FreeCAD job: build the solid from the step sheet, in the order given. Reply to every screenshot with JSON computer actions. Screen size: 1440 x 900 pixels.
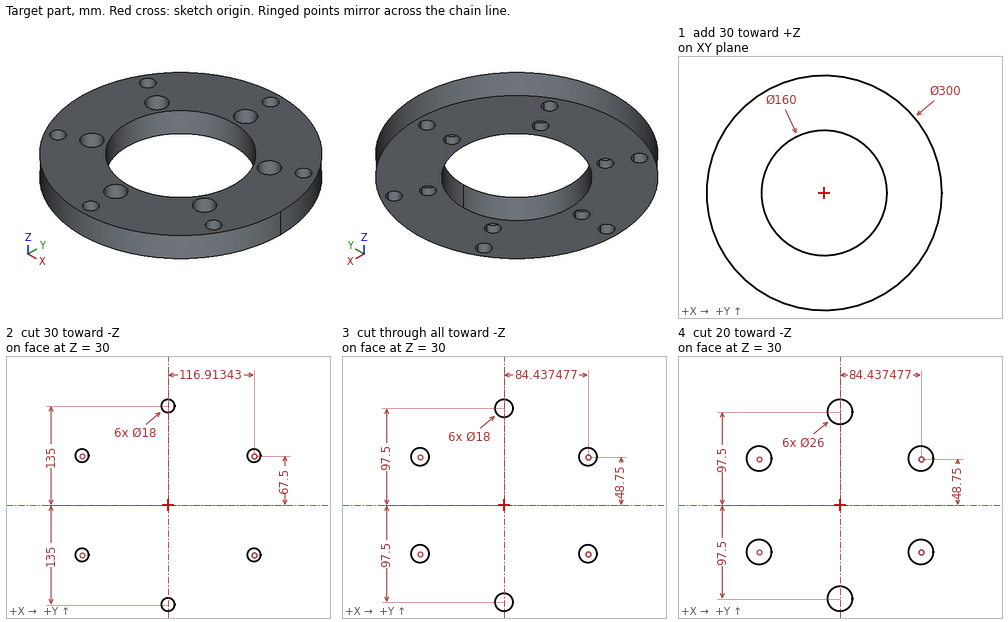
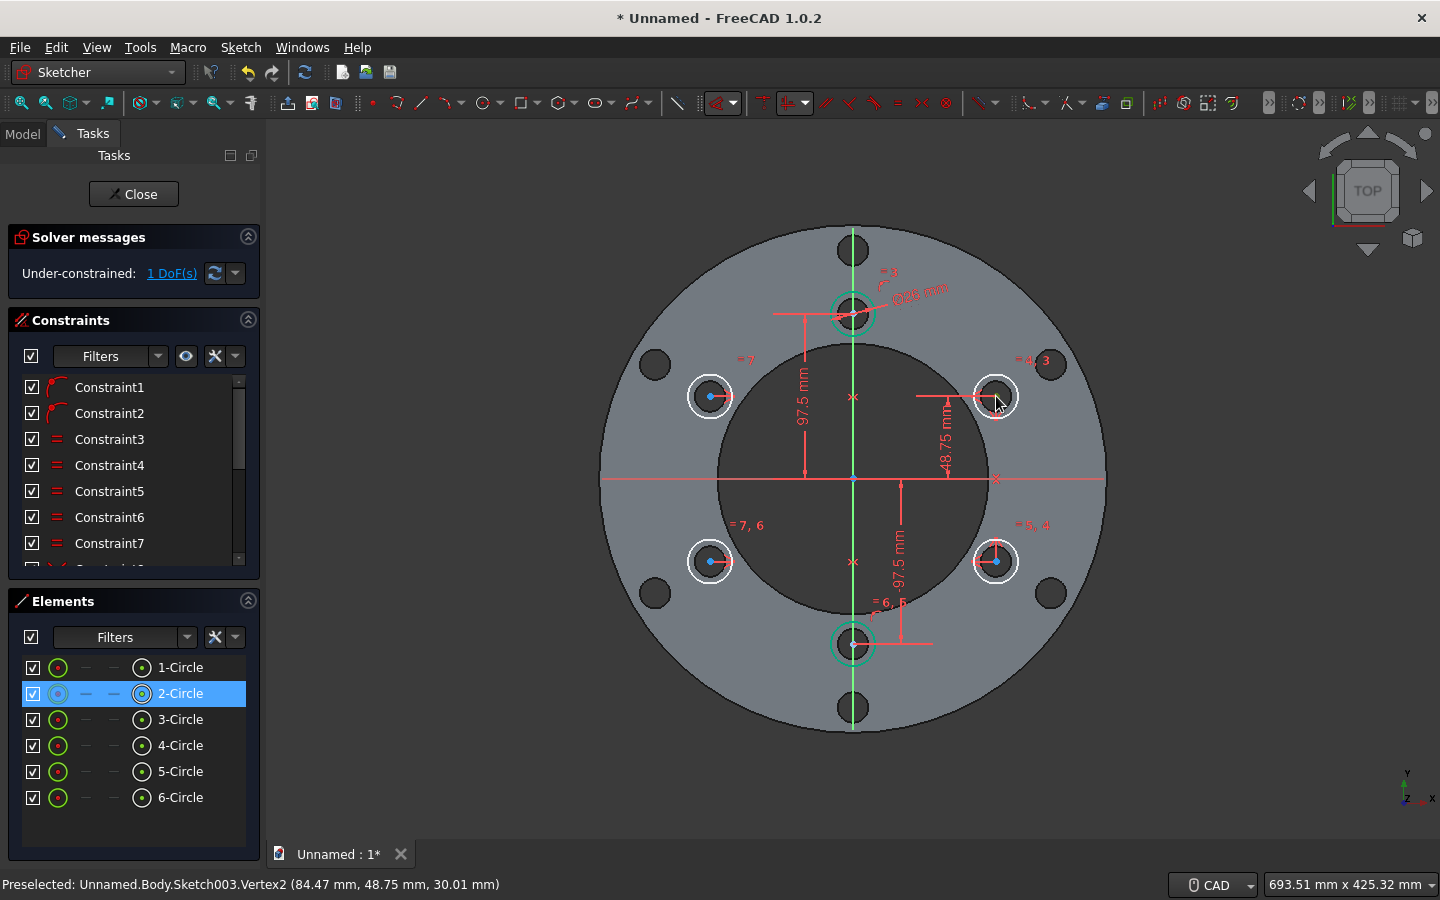
{"action": "key", "text": "l"}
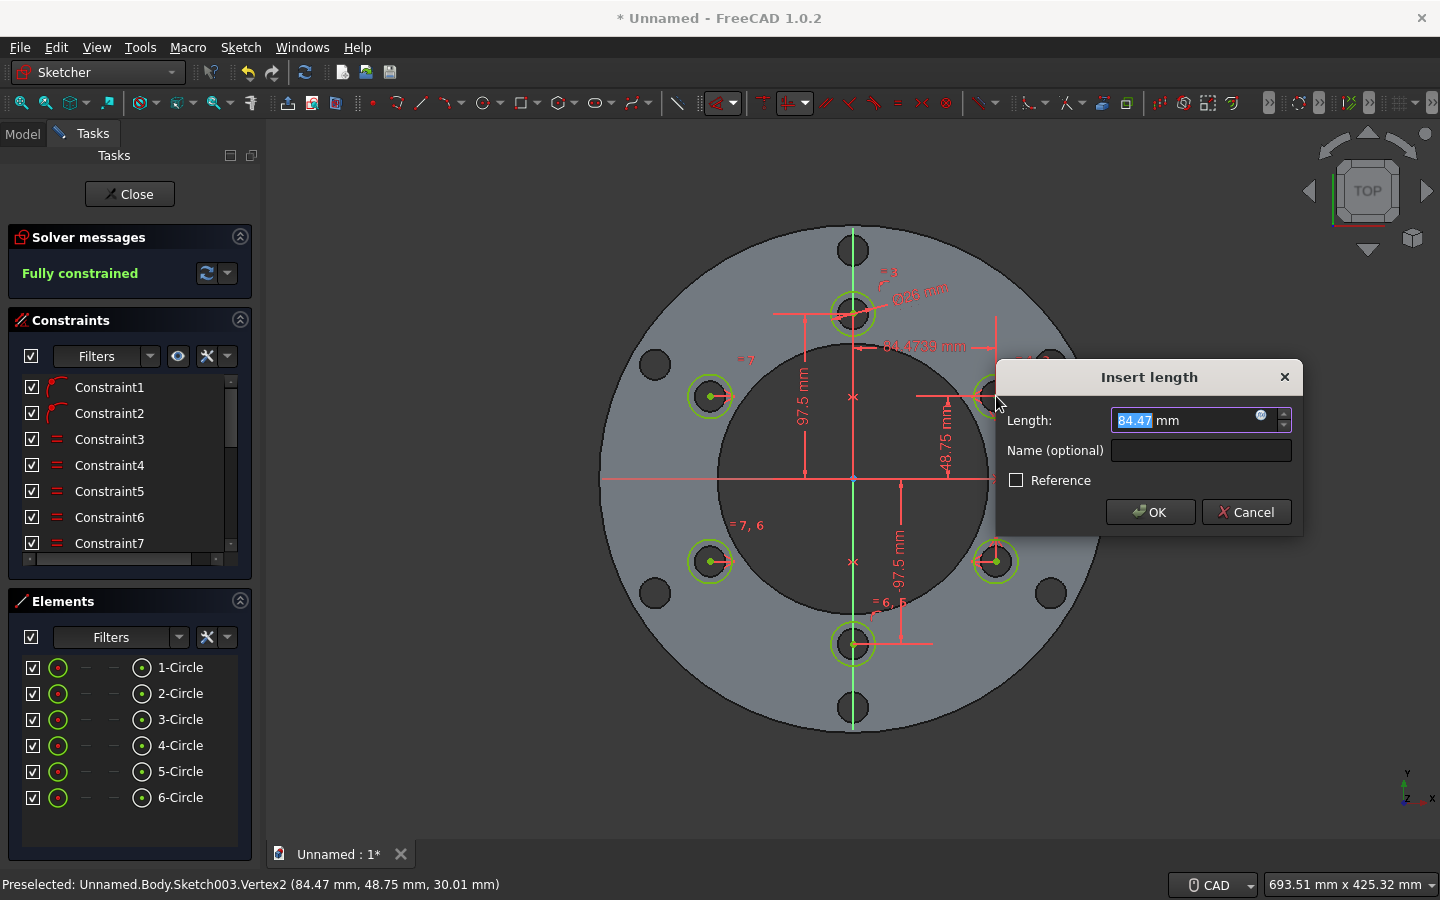
{"action": "type", "text": "84.437477"}
{"action": "key", "text": "Return"}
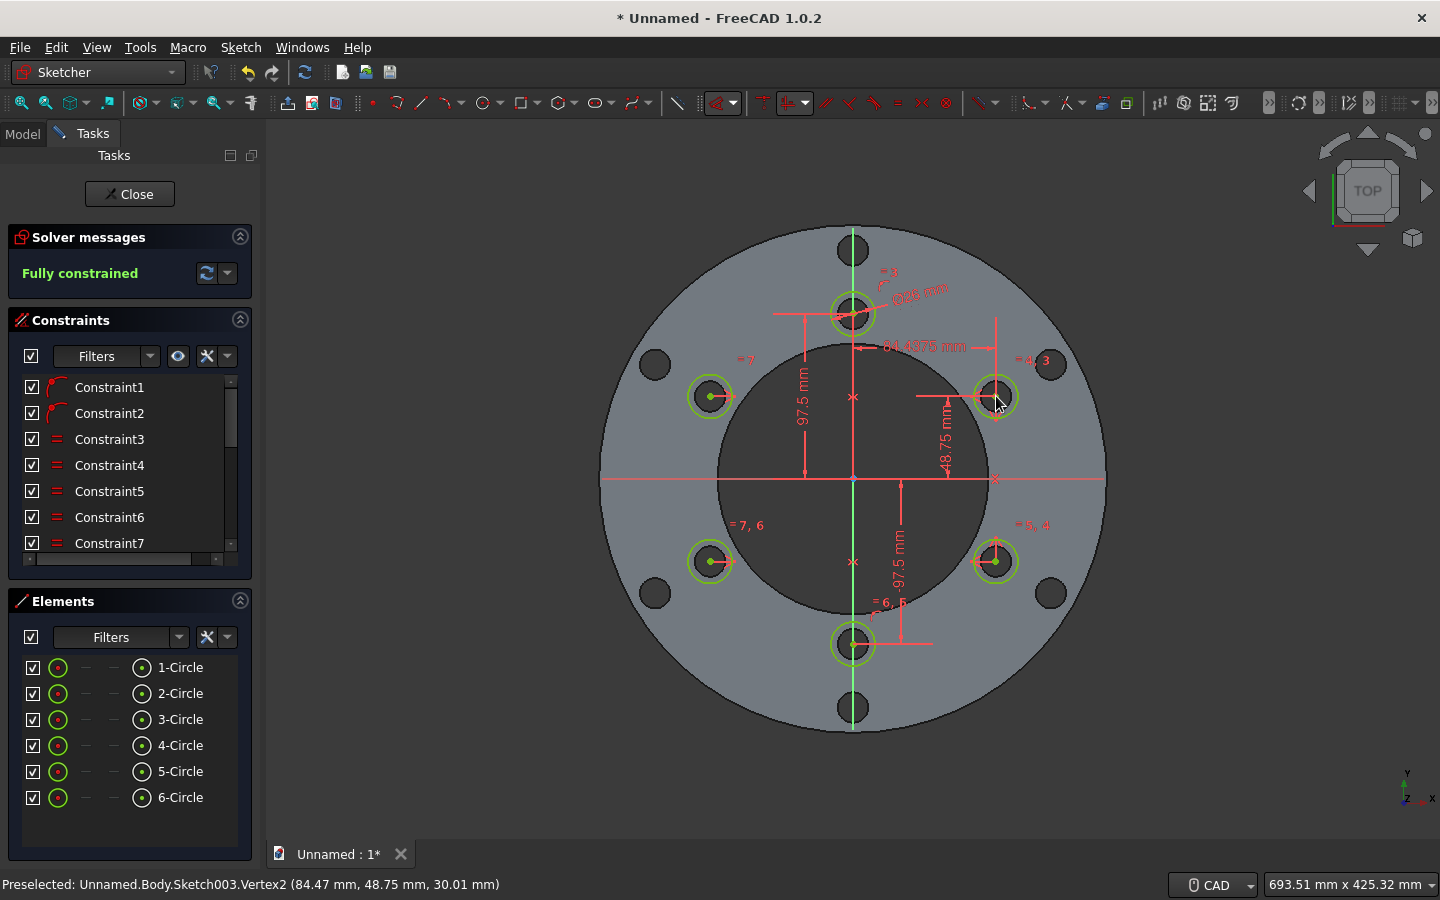
{"action": "left_click", "coordinate": [130, 194]}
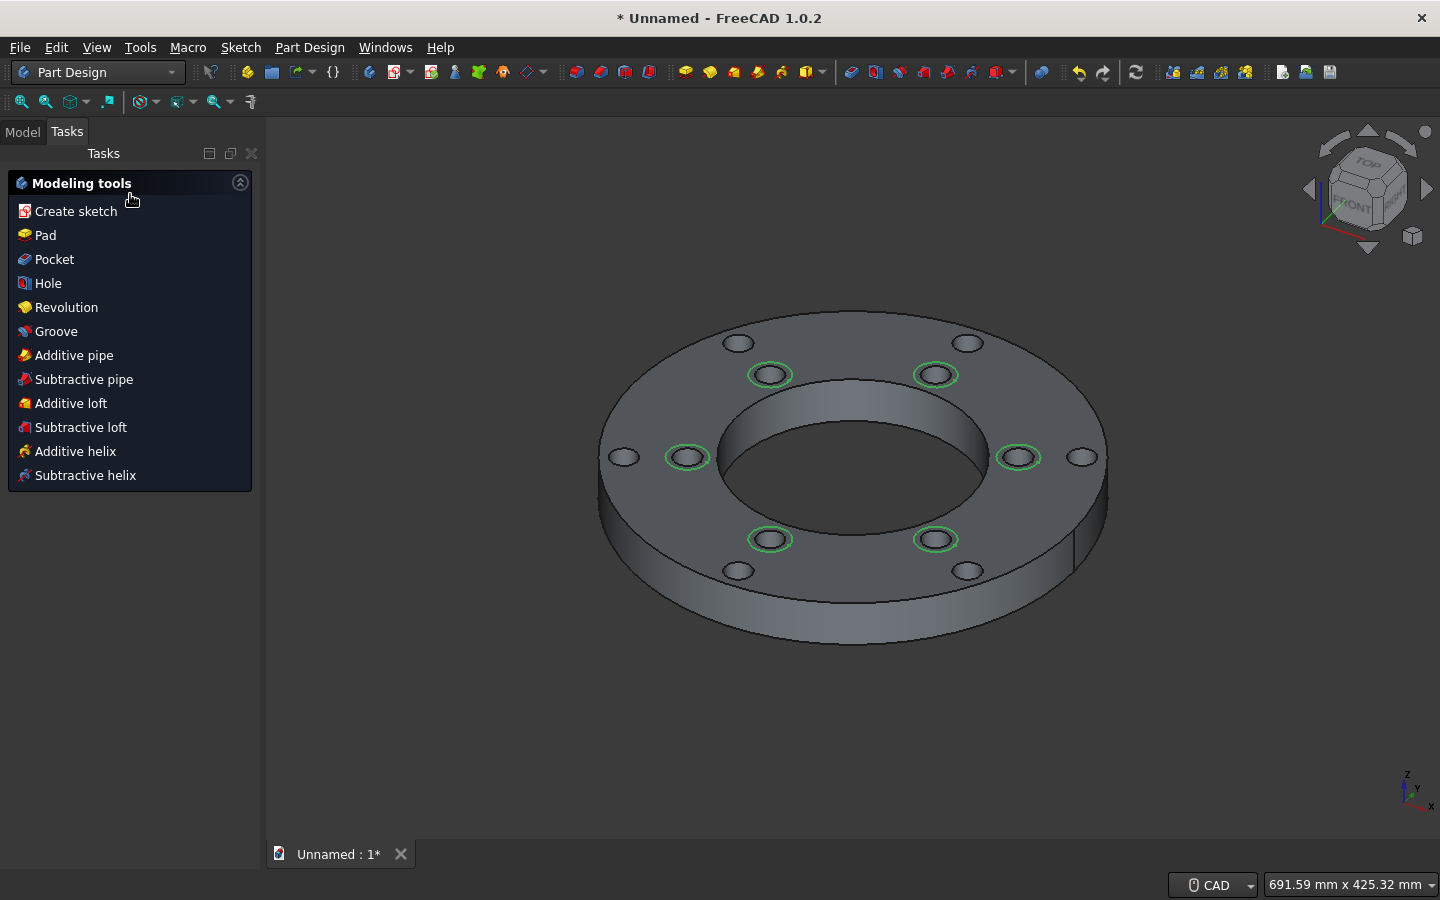
{"action": "left_click", "coordinate": [852, 72]}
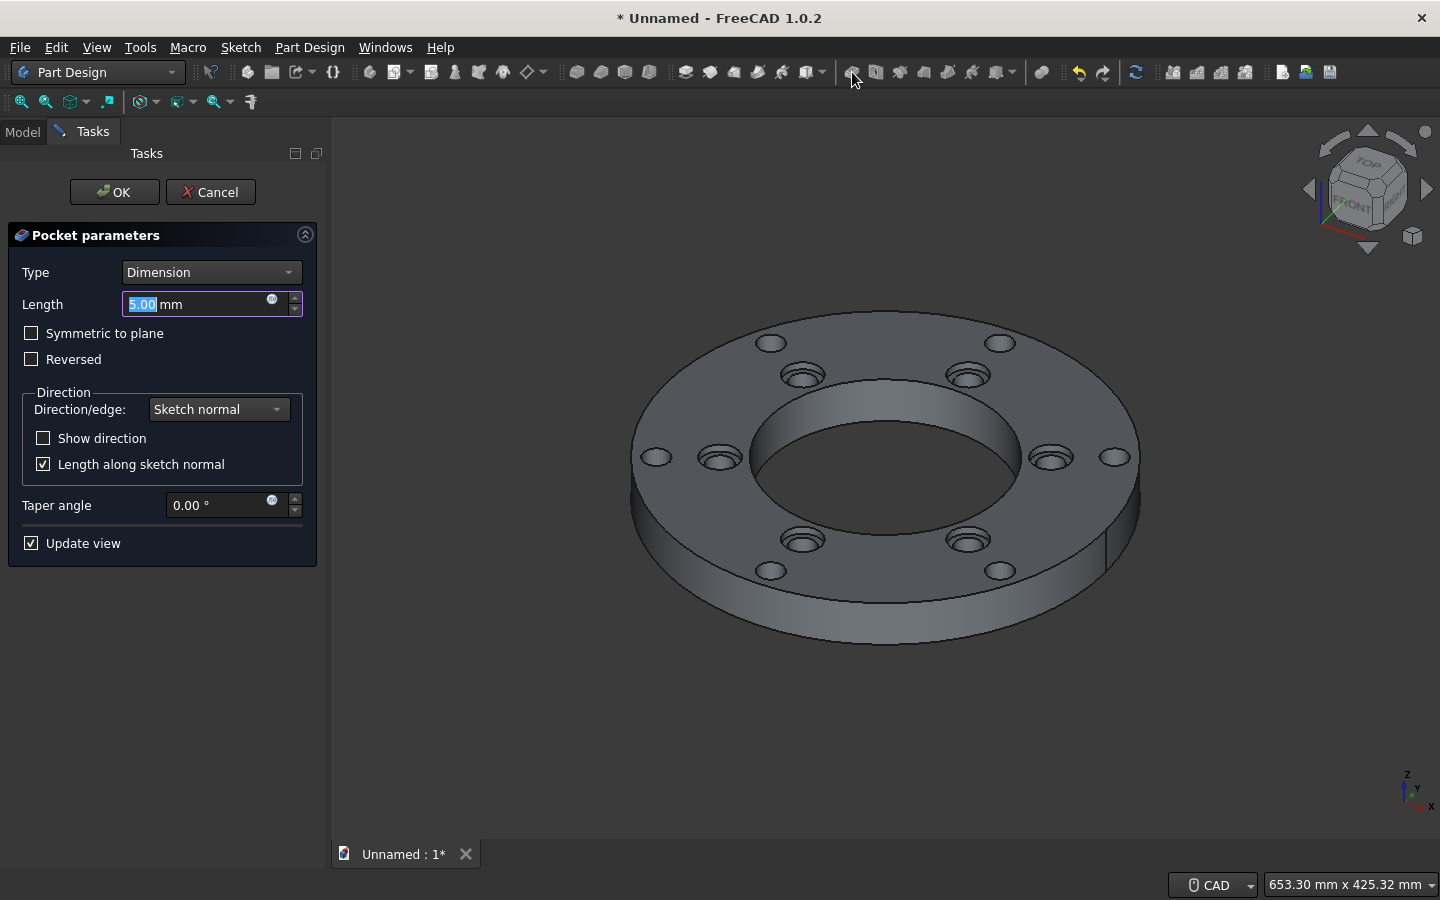
{"action": "type", "text": "20"}
{"action": "key", "text": "Tab"}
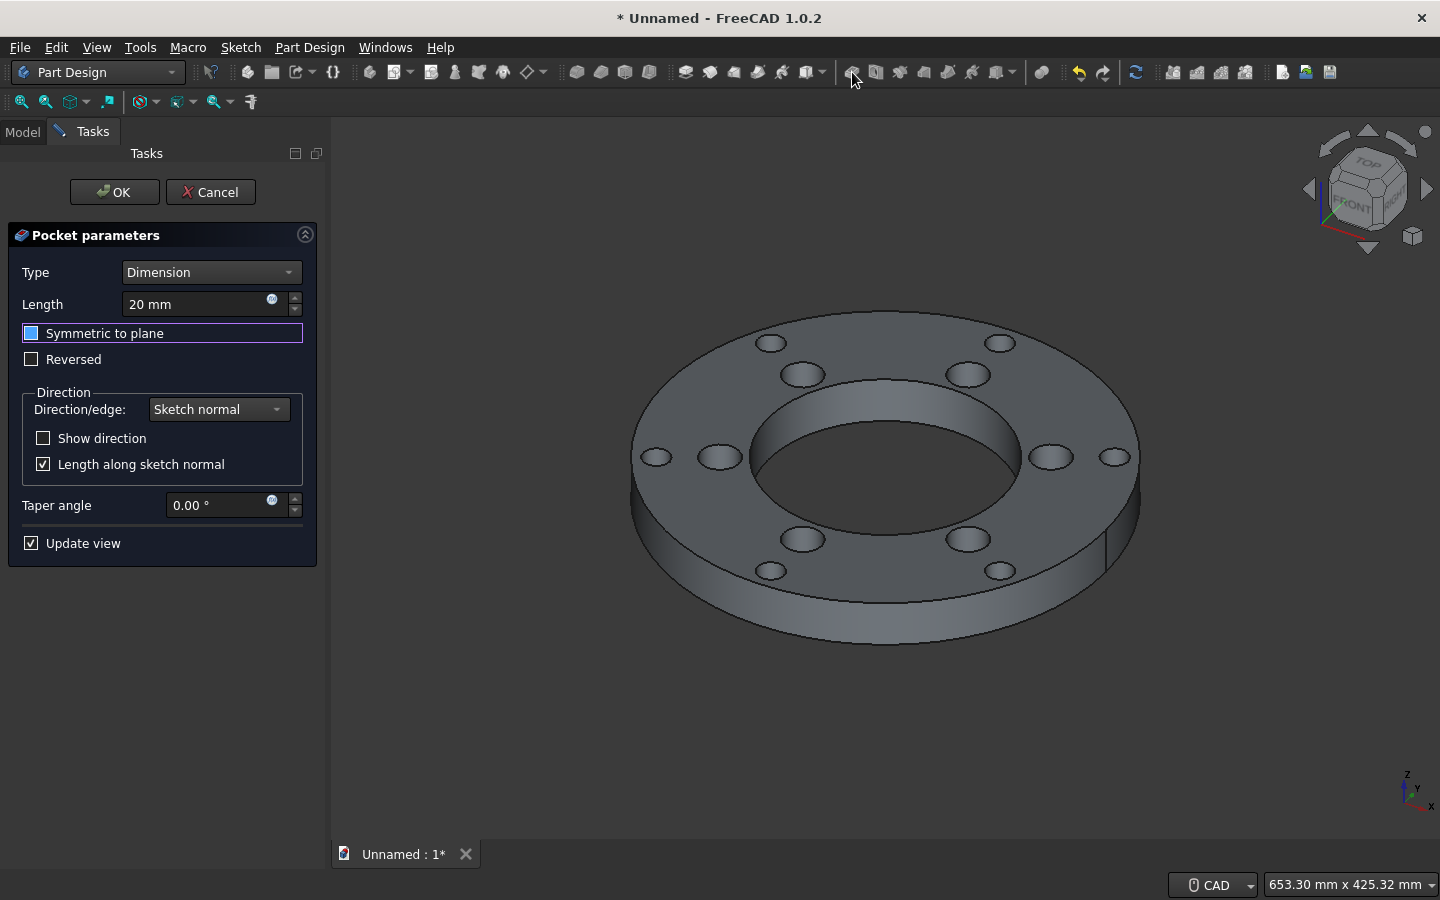
{"action": "left_click", "coordinate": [115, 192]}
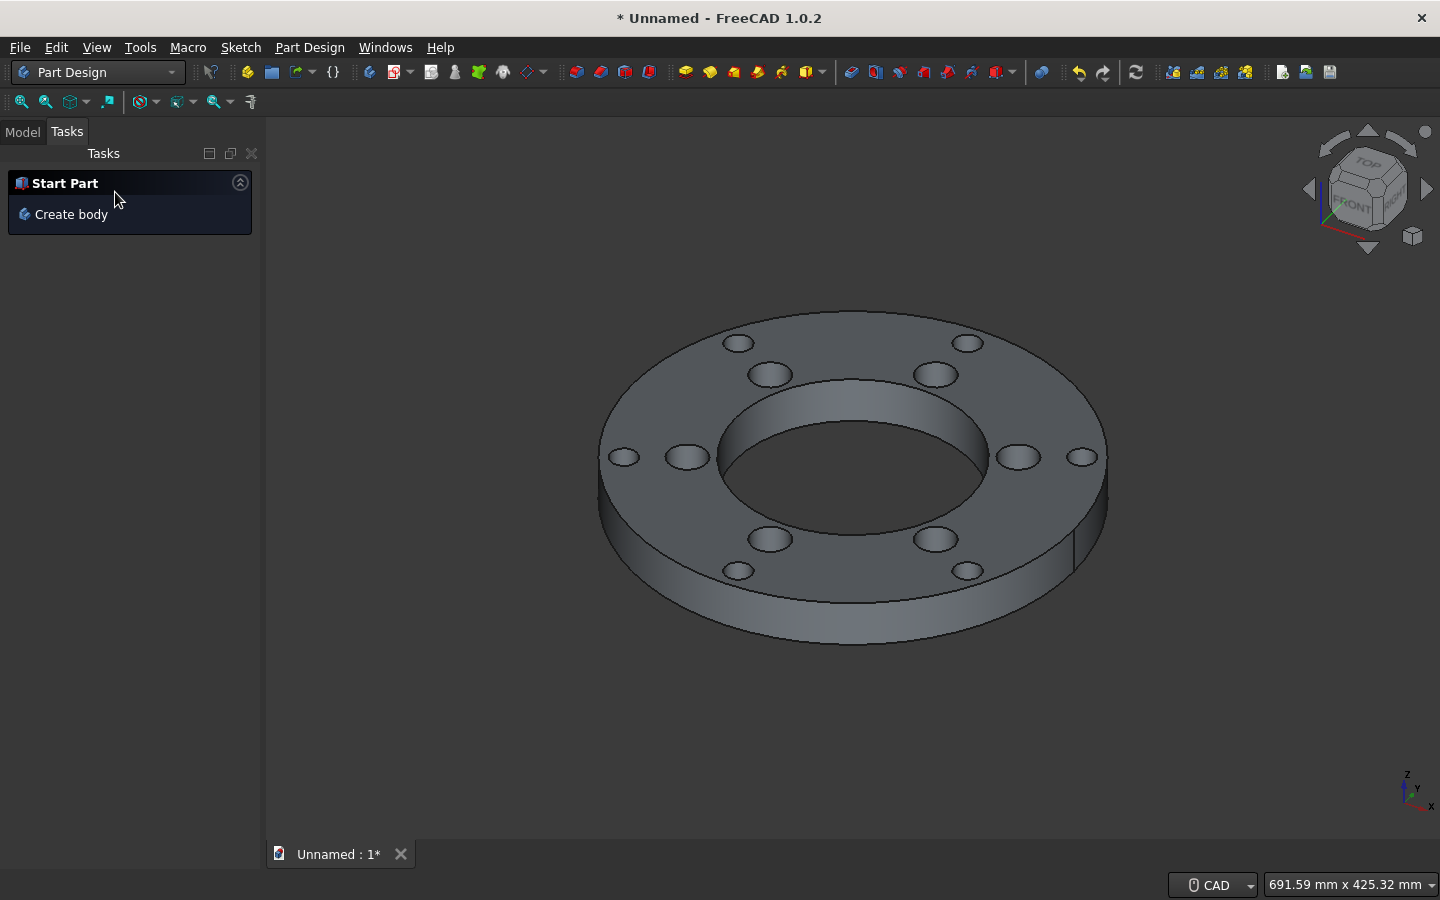
{"action": "key", "text": "0"}